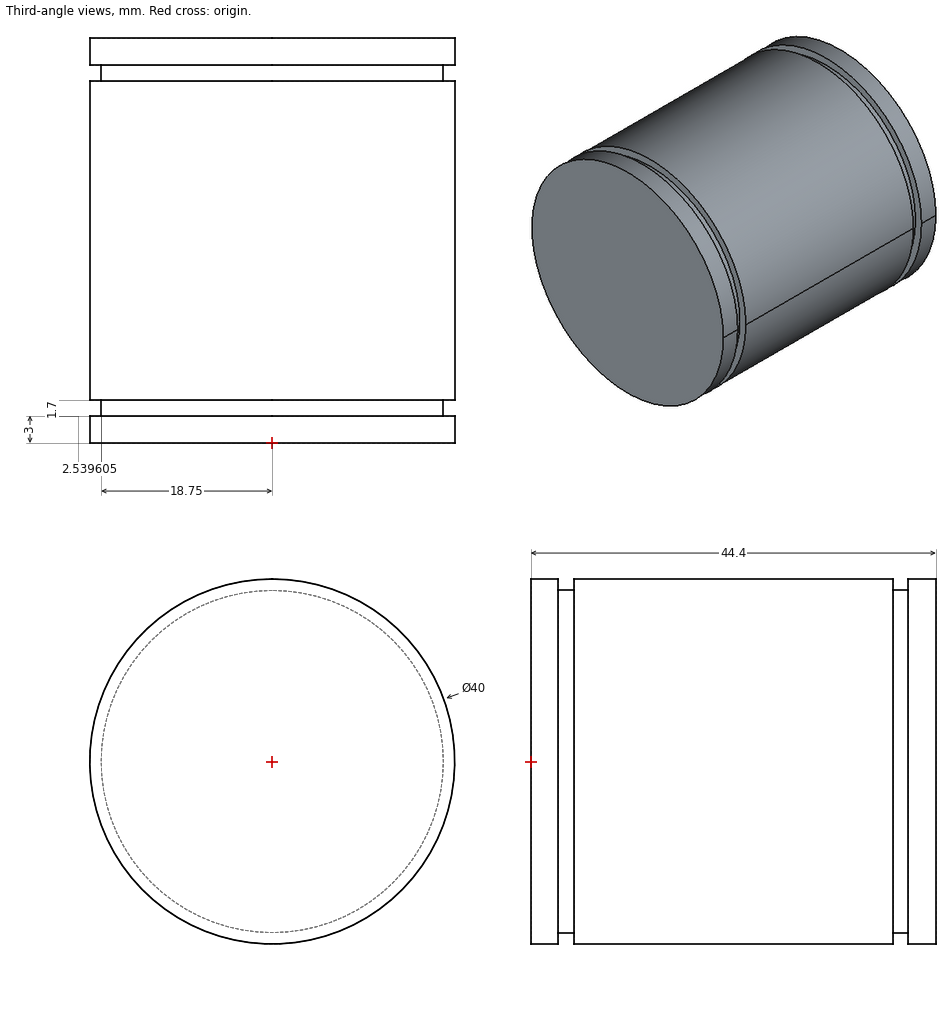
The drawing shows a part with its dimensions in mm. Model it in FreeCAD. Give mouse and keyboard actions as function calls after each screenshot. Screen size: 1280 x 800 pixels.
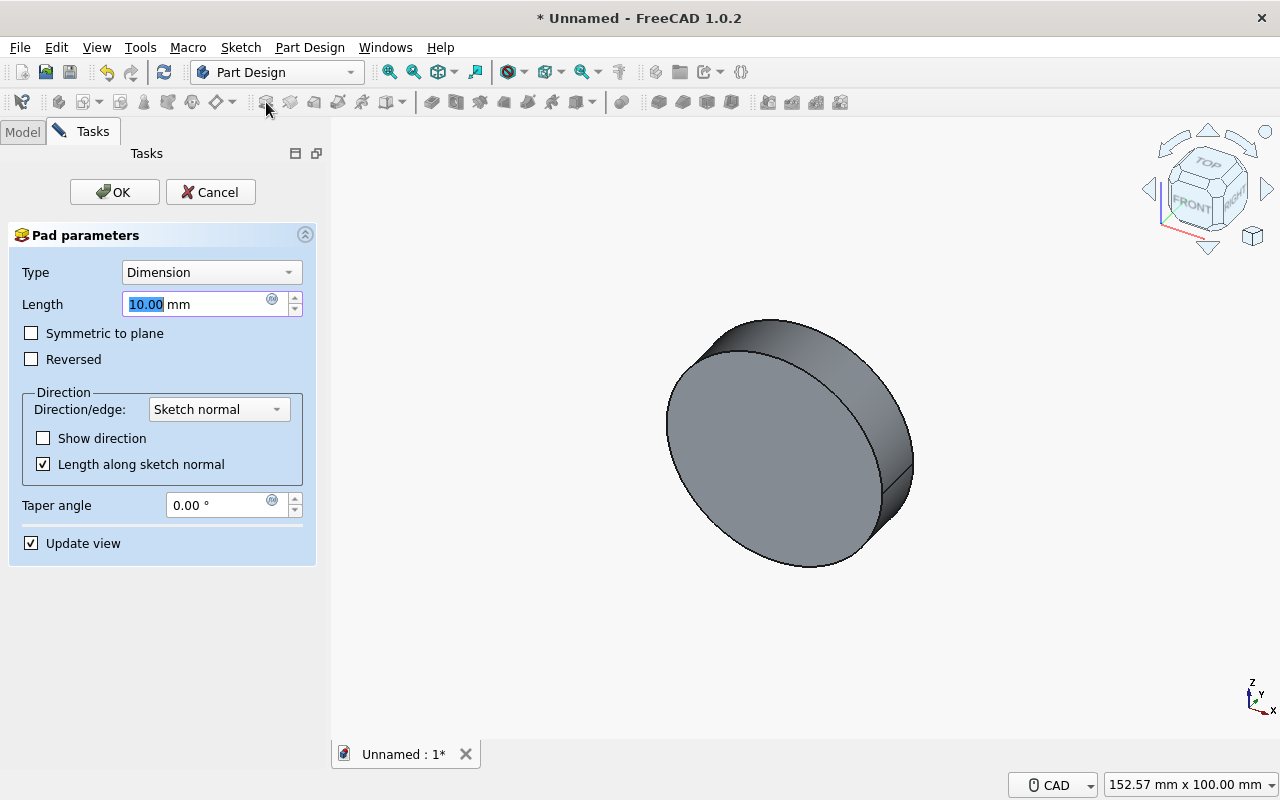
text(44.4)
key(Tab)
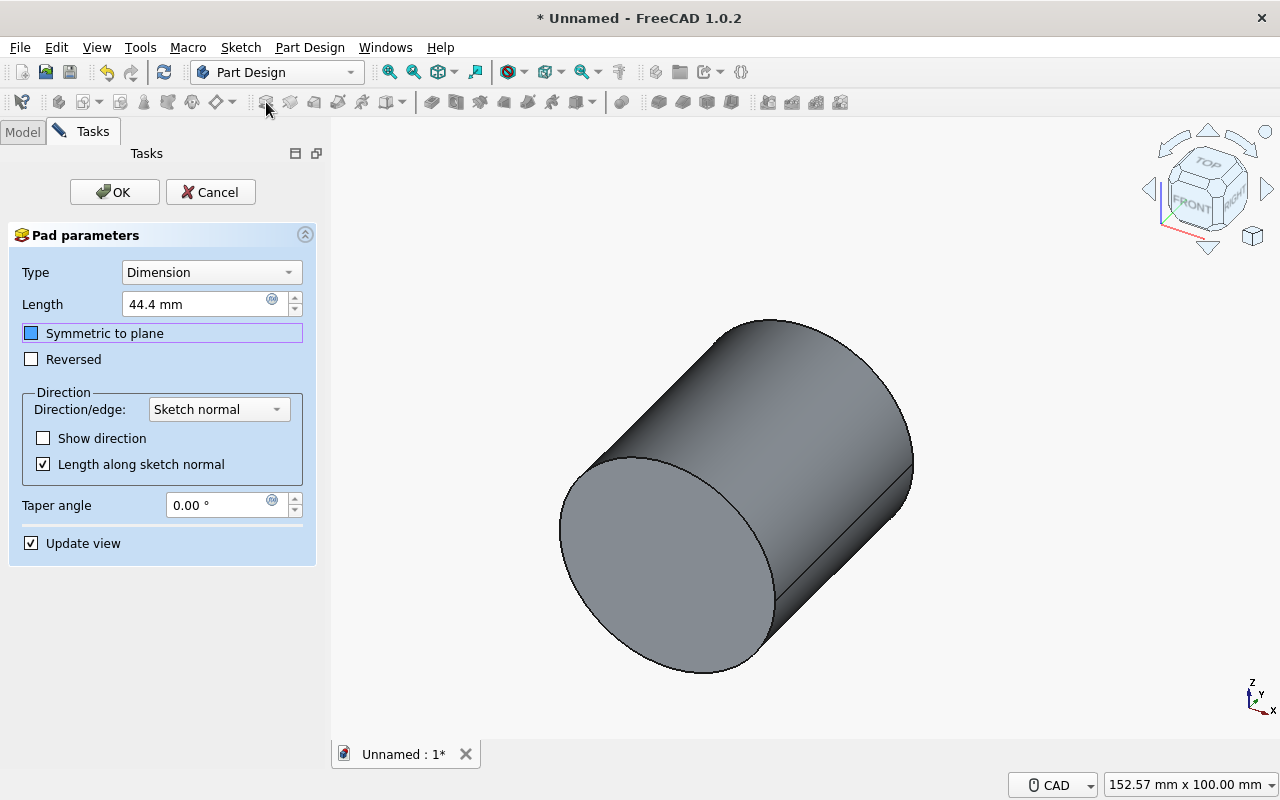
click(30, 359)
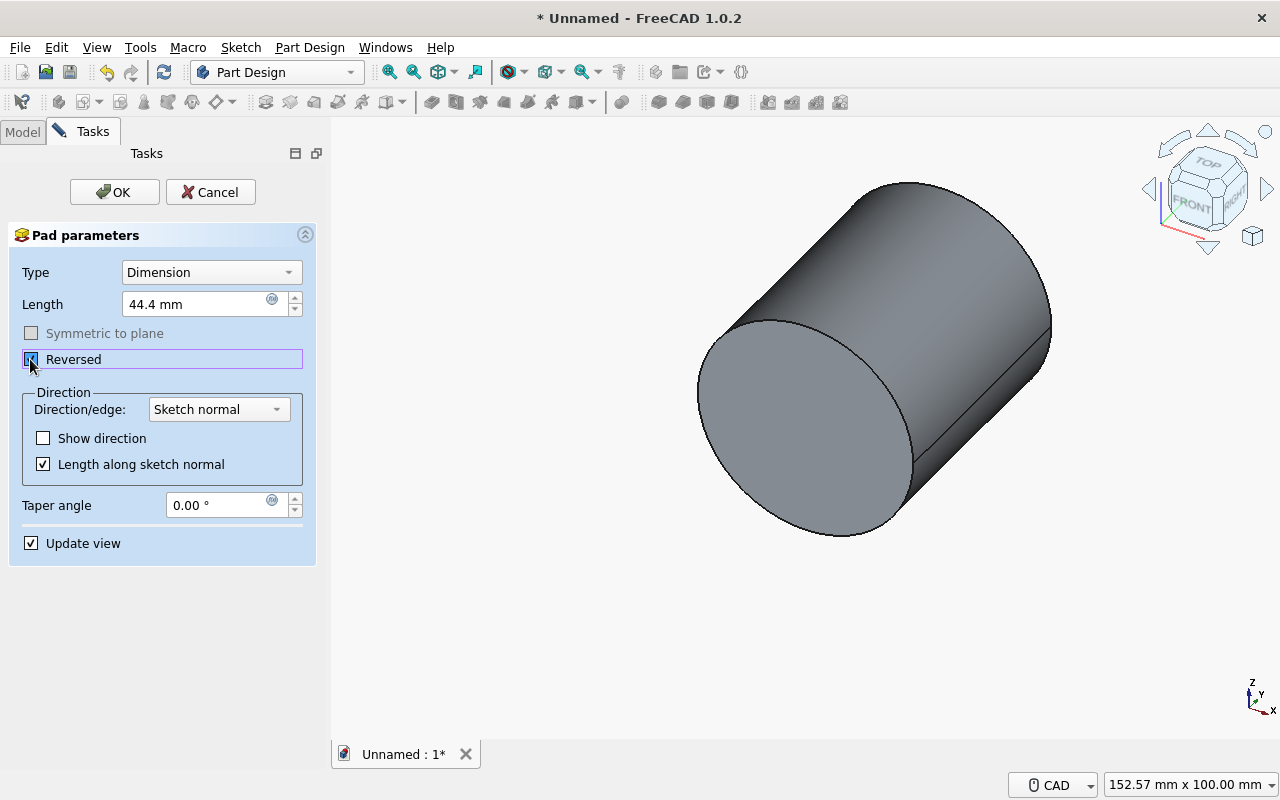
click(115, 192)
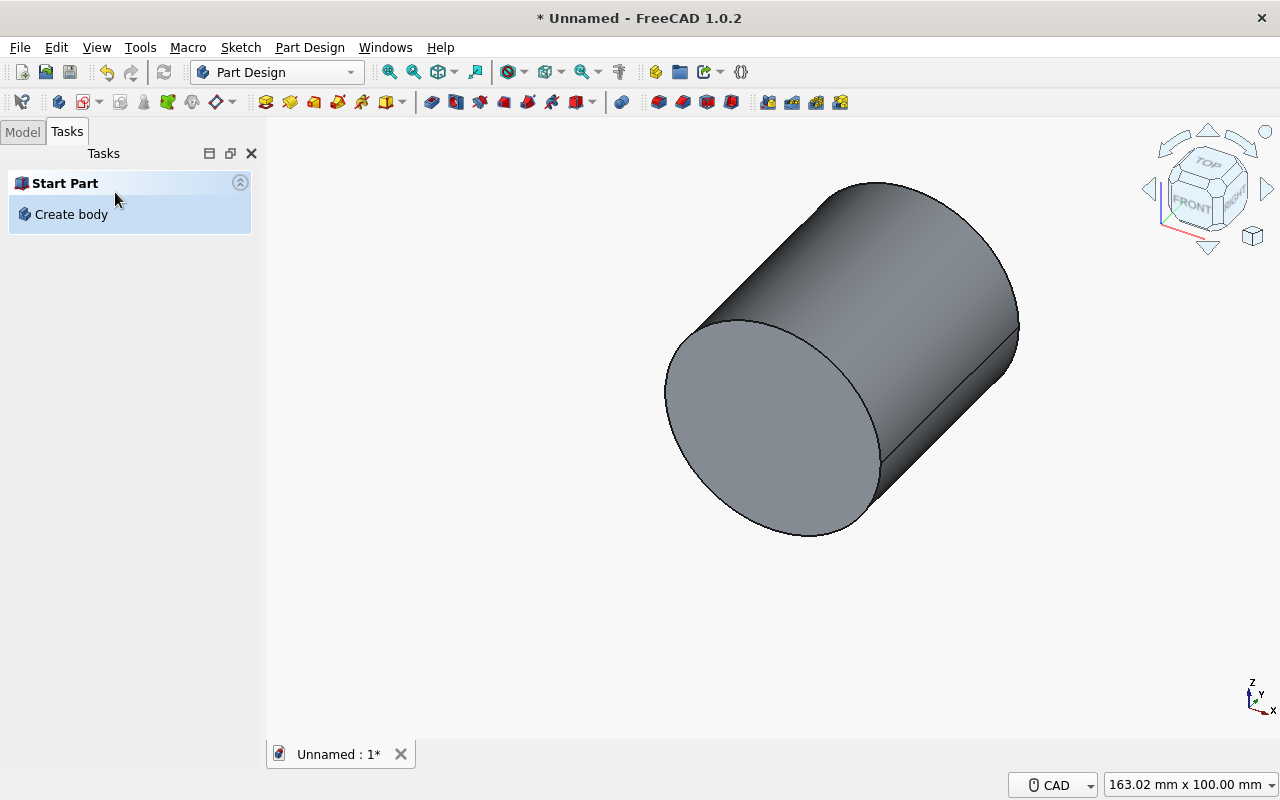
click(84, 102)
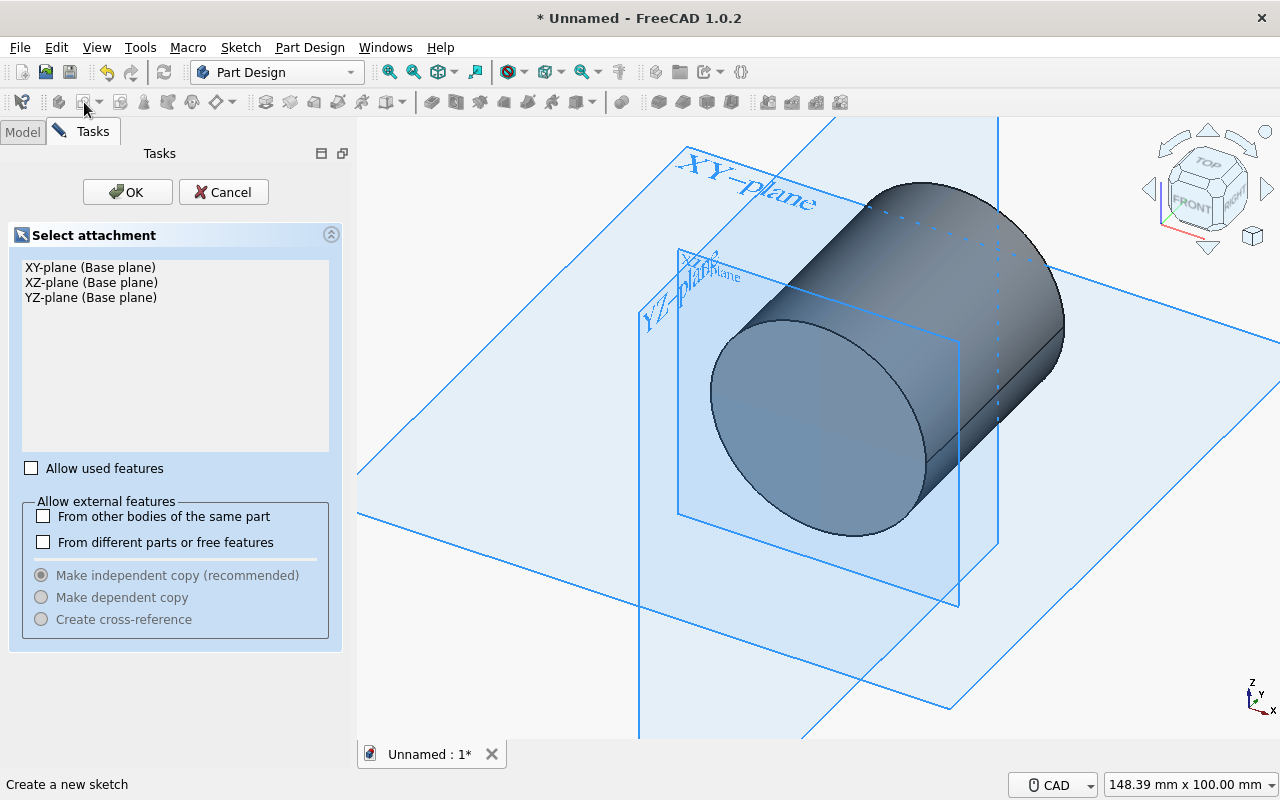
click(82, 268)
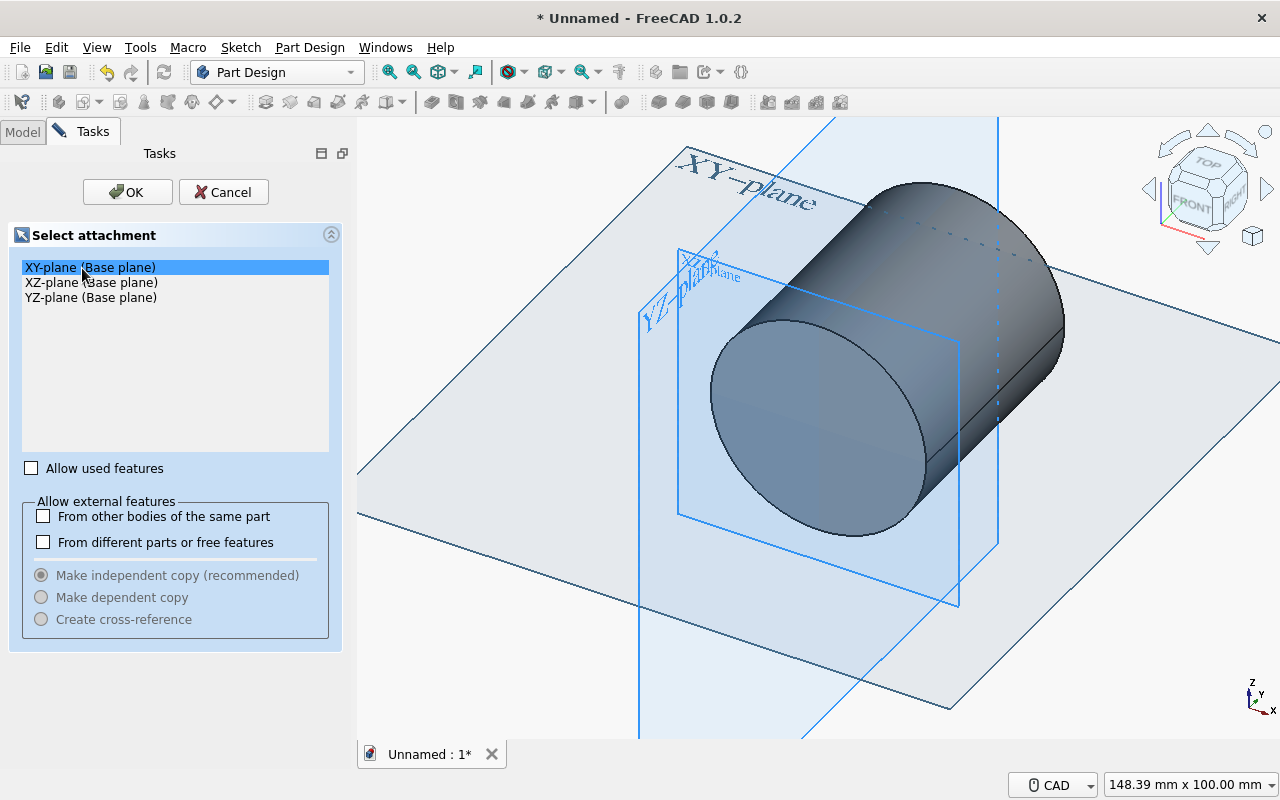
click(128, 192)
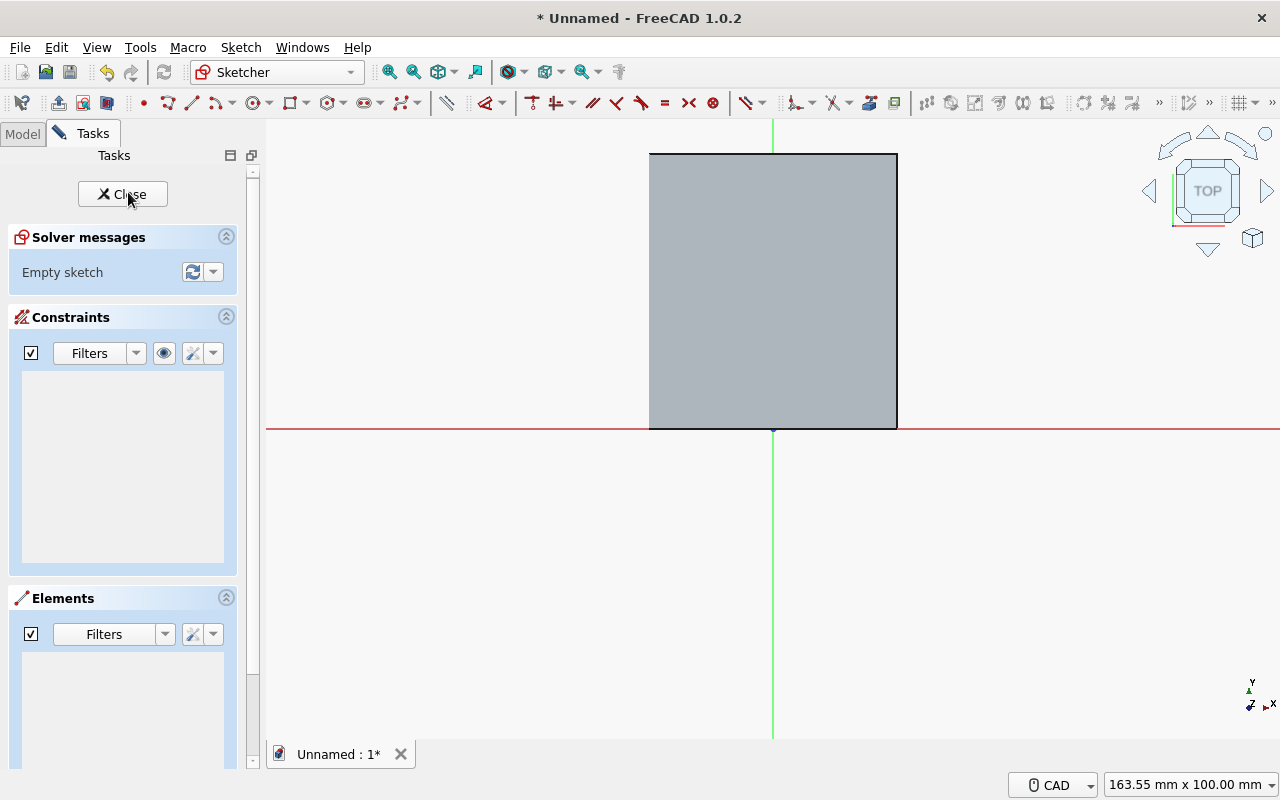
key(q)
key(s)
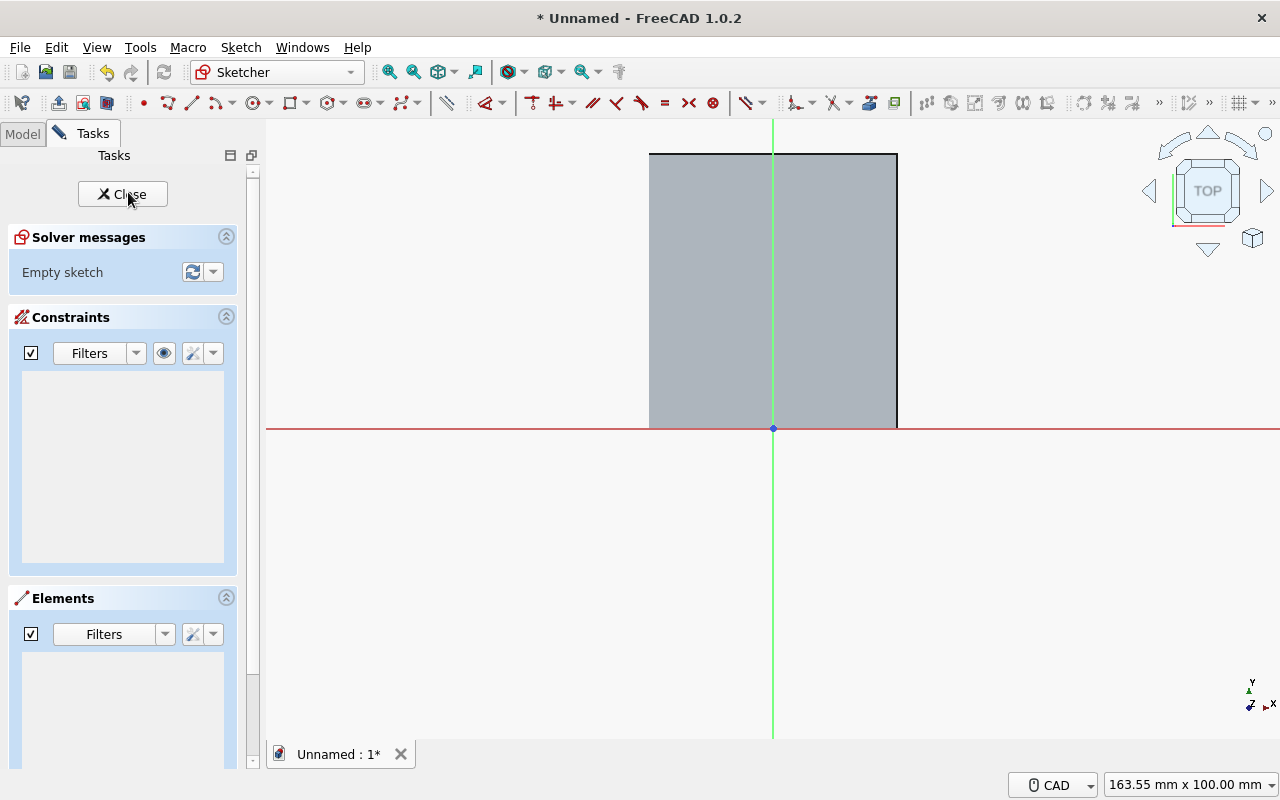
scroll(646, 404, up, 15)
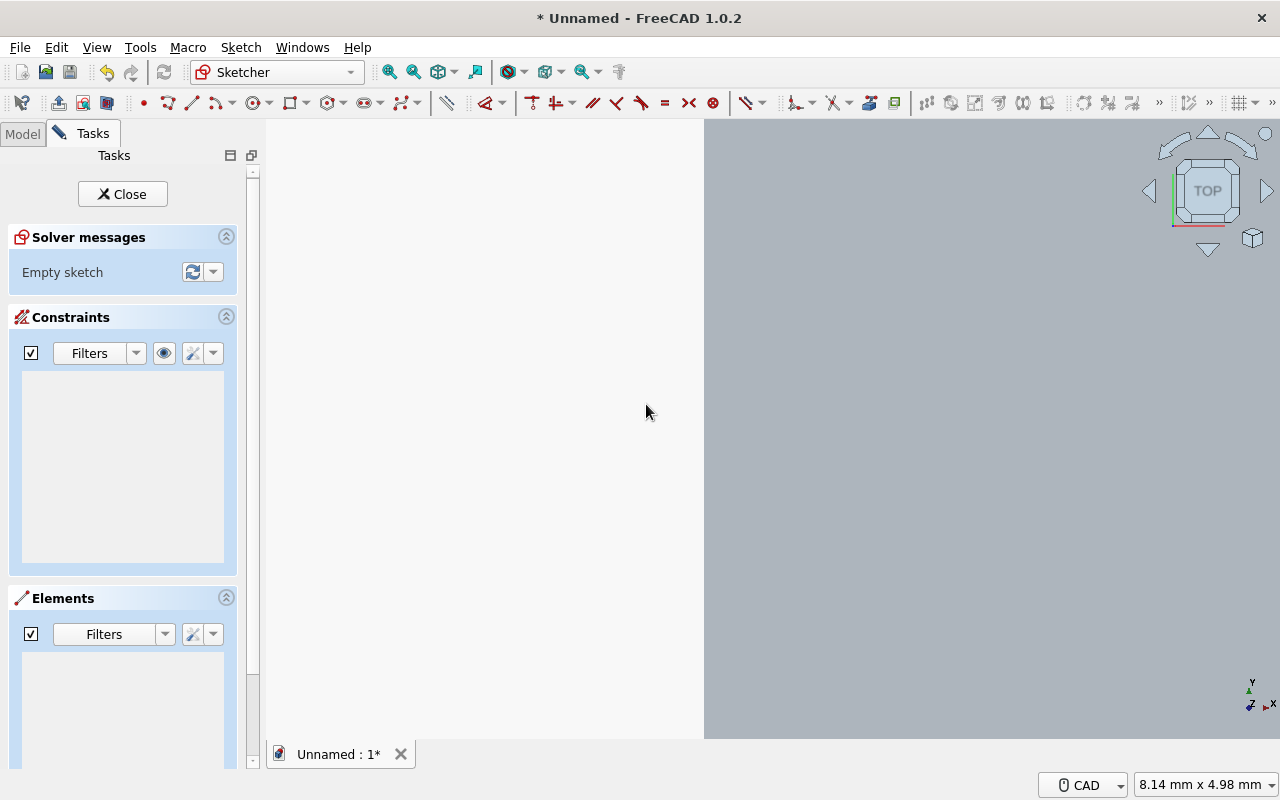
scroll(687, 404, up, 3)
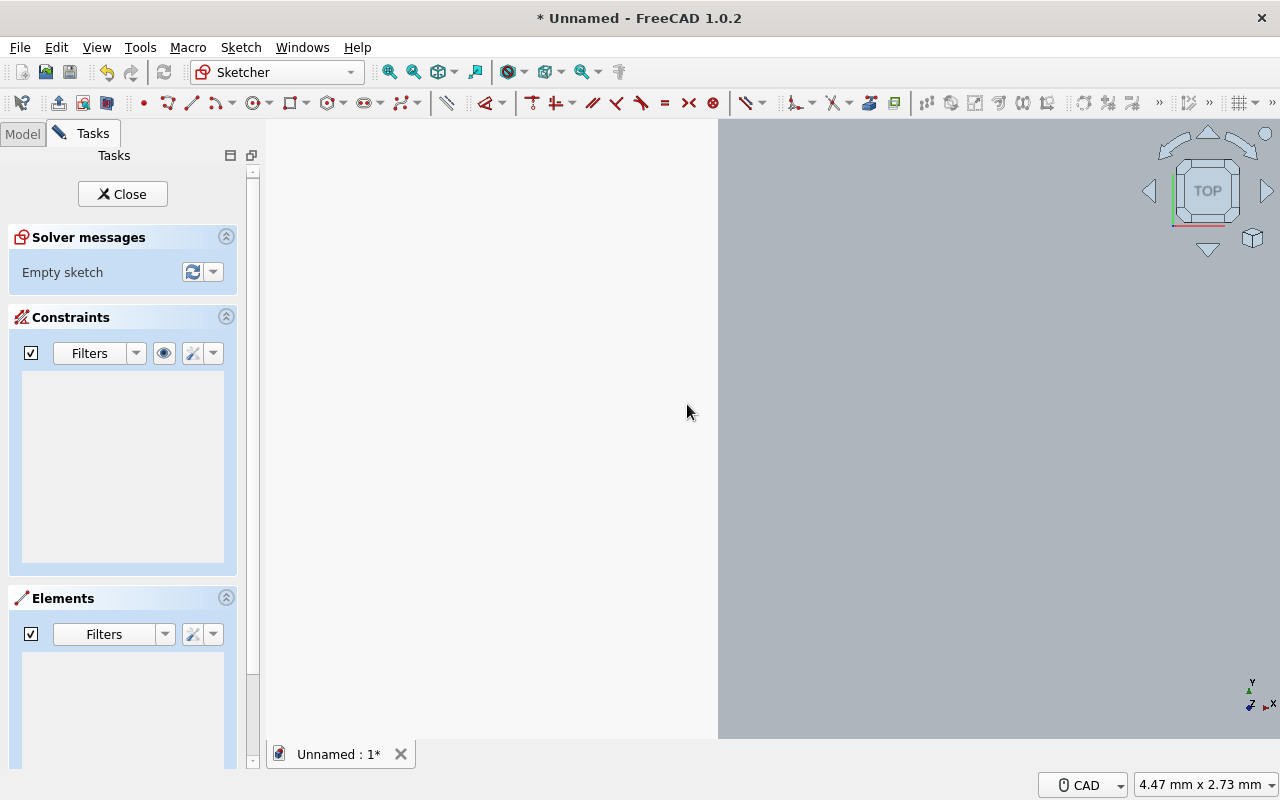
click(290, 104)